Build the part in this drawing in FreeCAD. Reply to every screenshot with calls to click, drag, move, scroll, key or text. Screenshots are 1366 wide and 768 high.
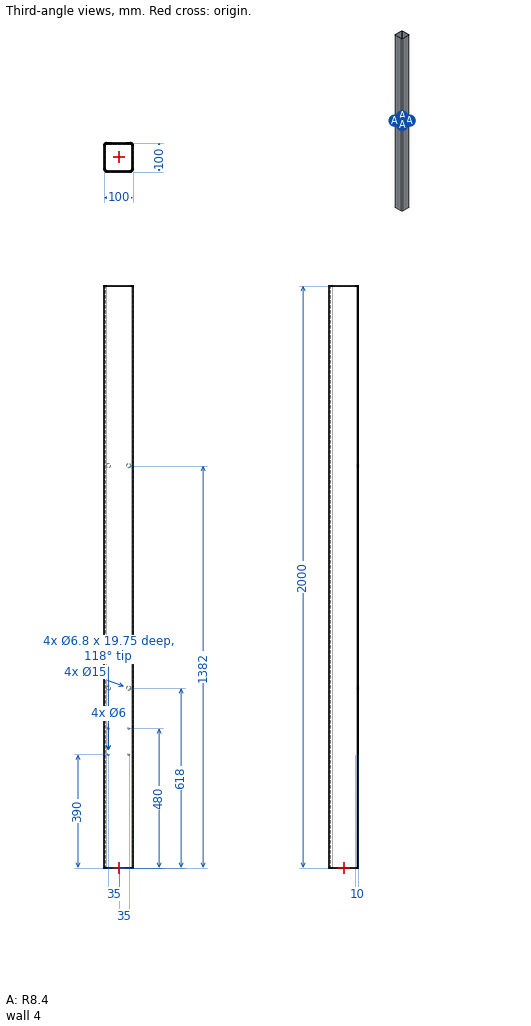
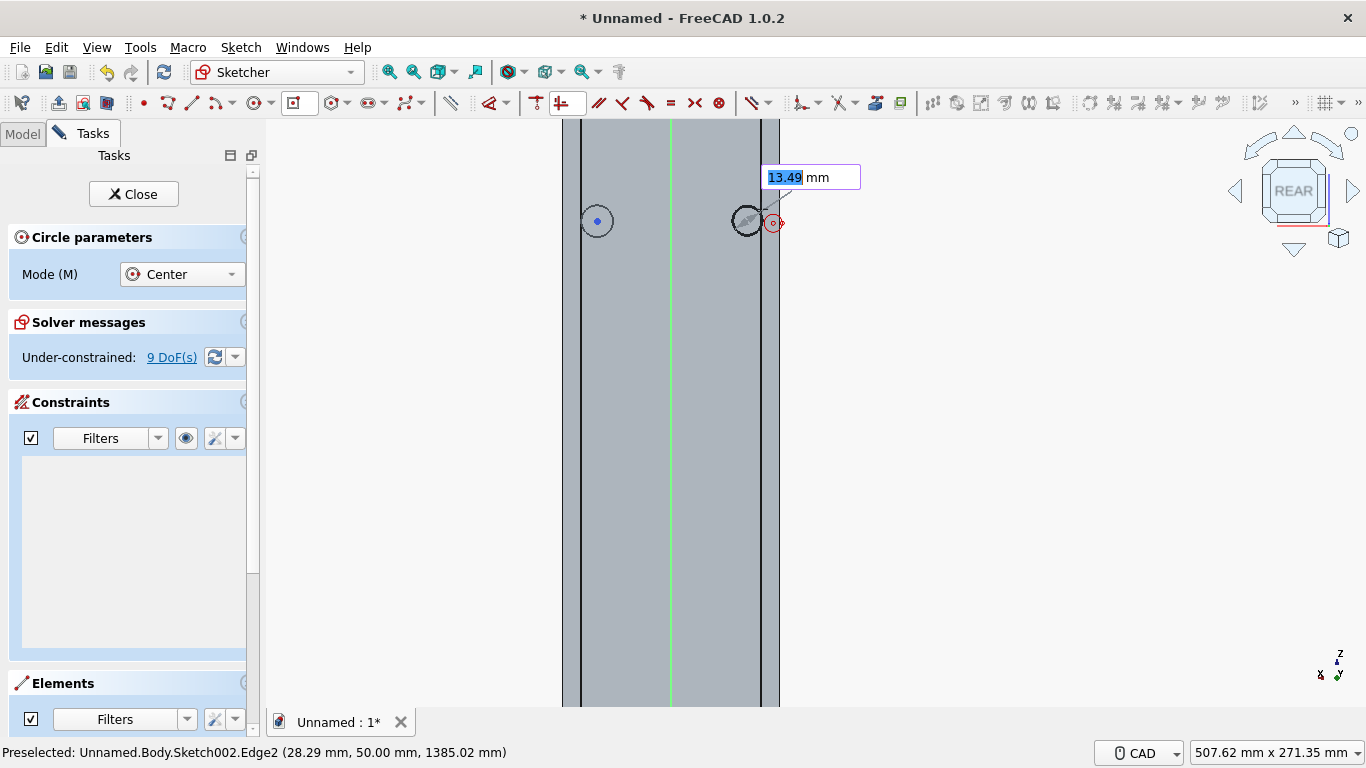
click(758, 207)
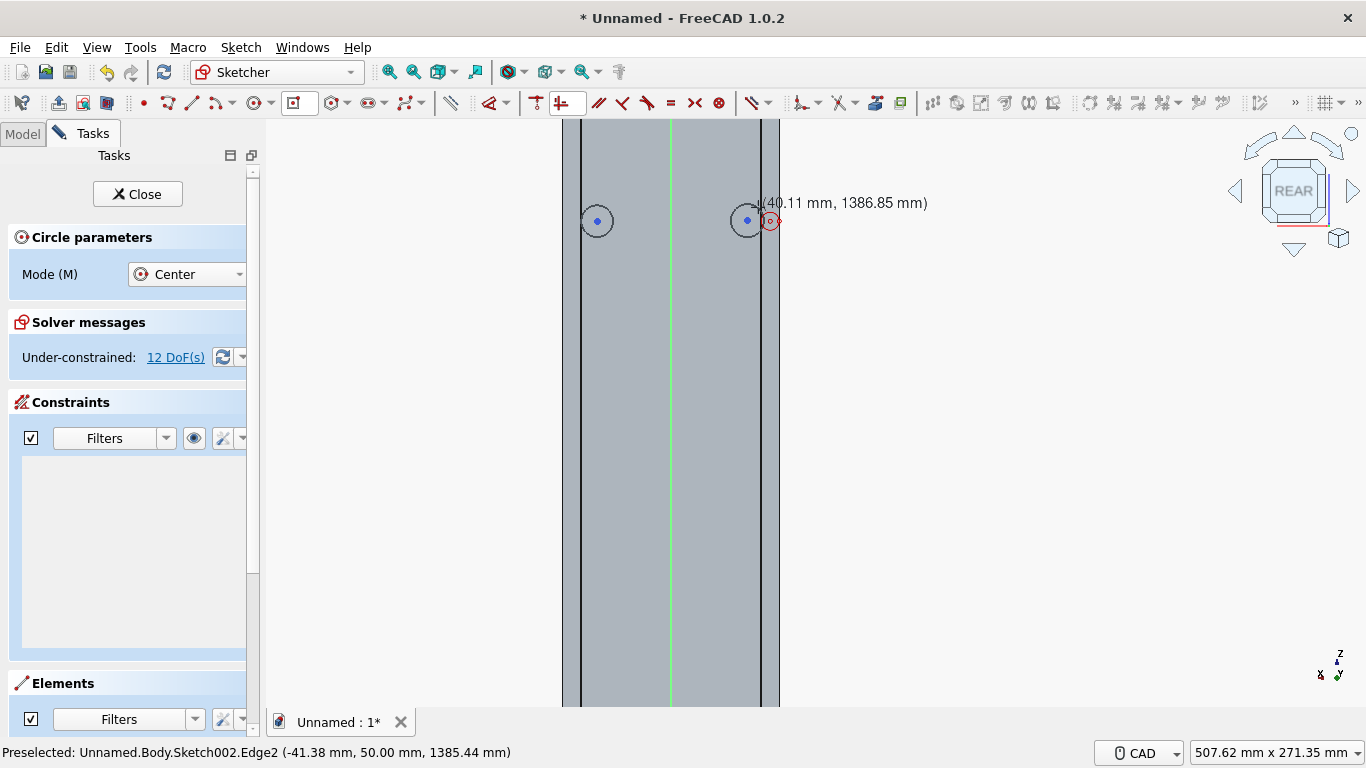
scroll(759, 210, down, 10)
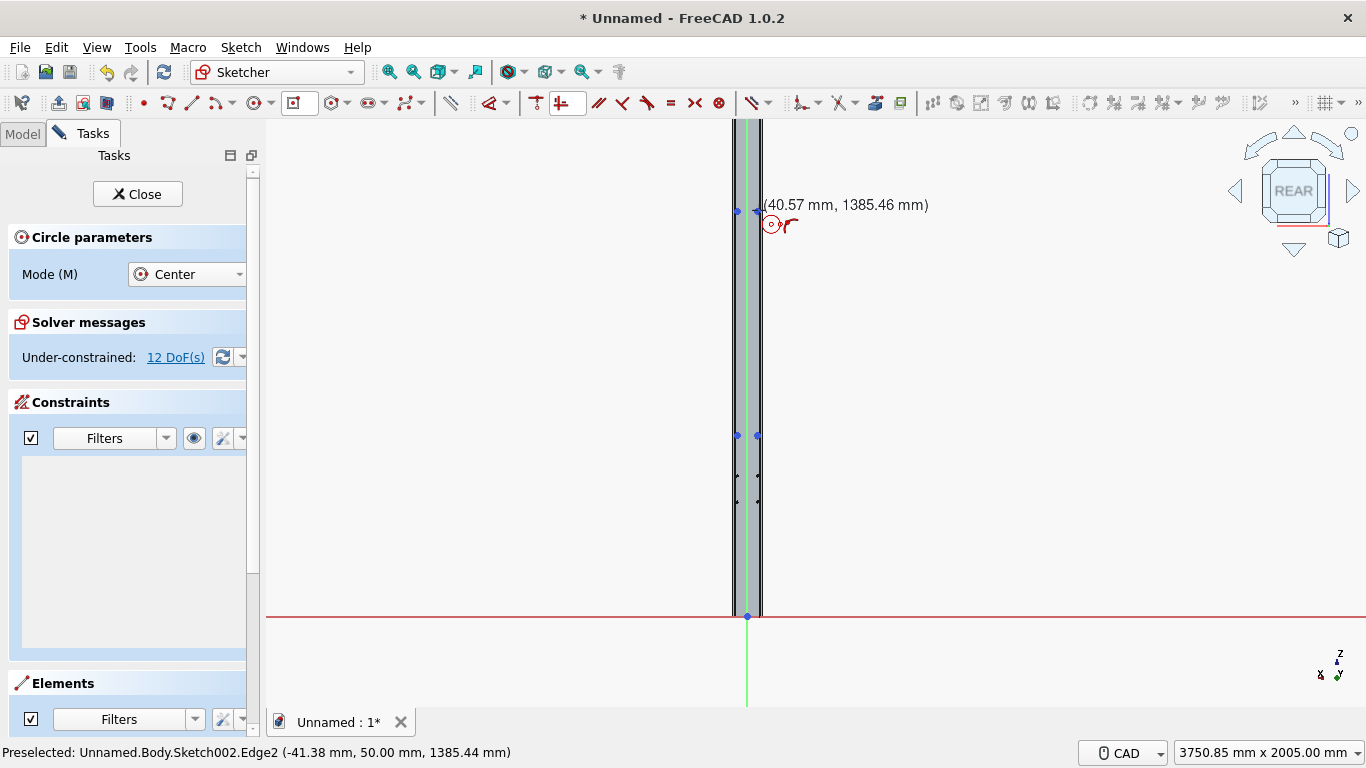
scroll(758, 502, up, 17)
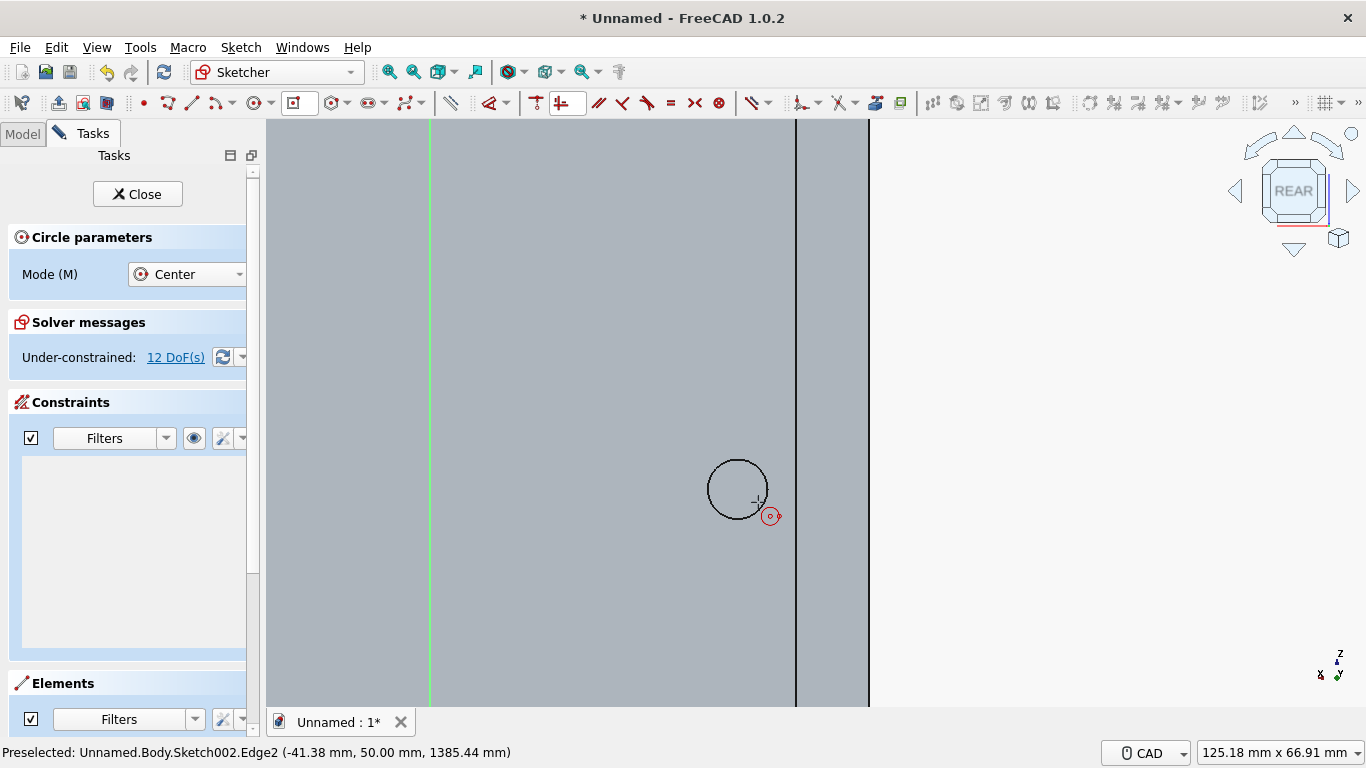
scroll(758, 503, down, 17)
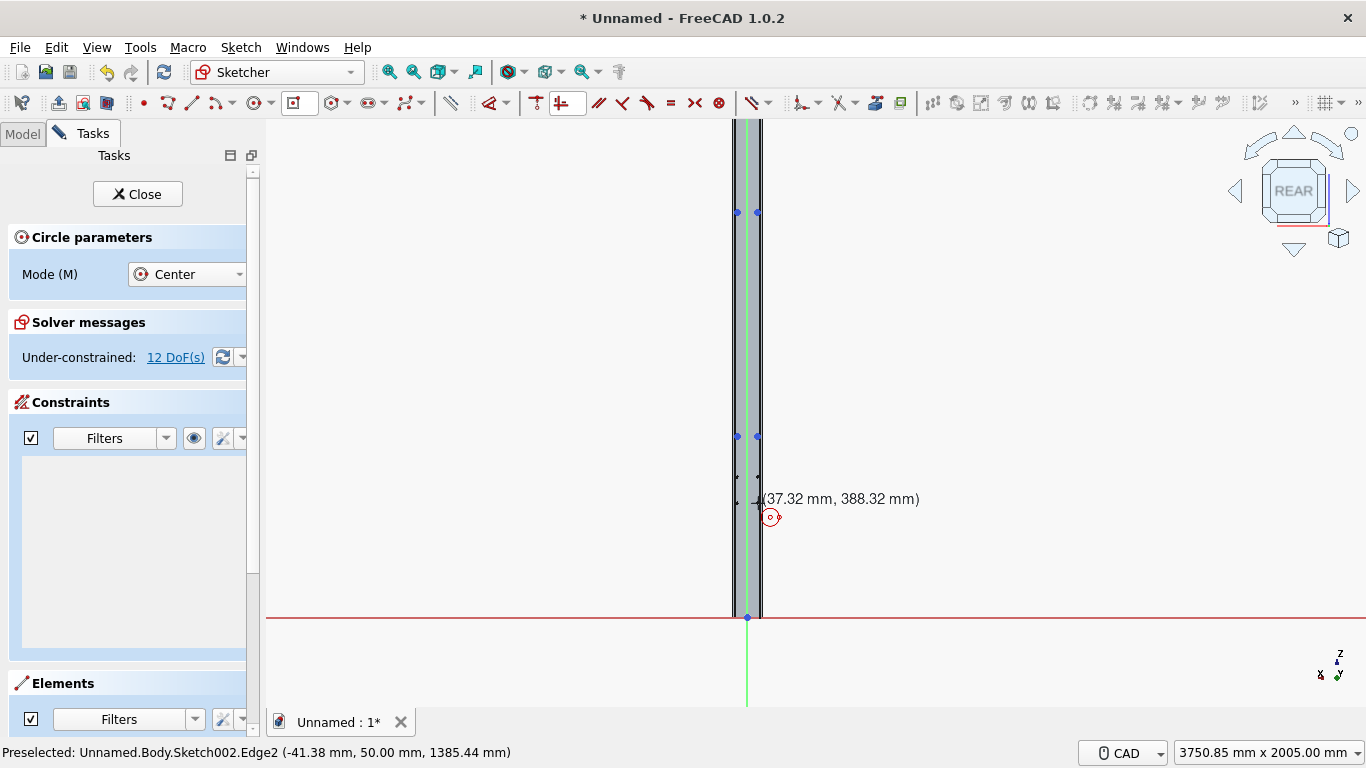
scroll(758, 503, up, 3)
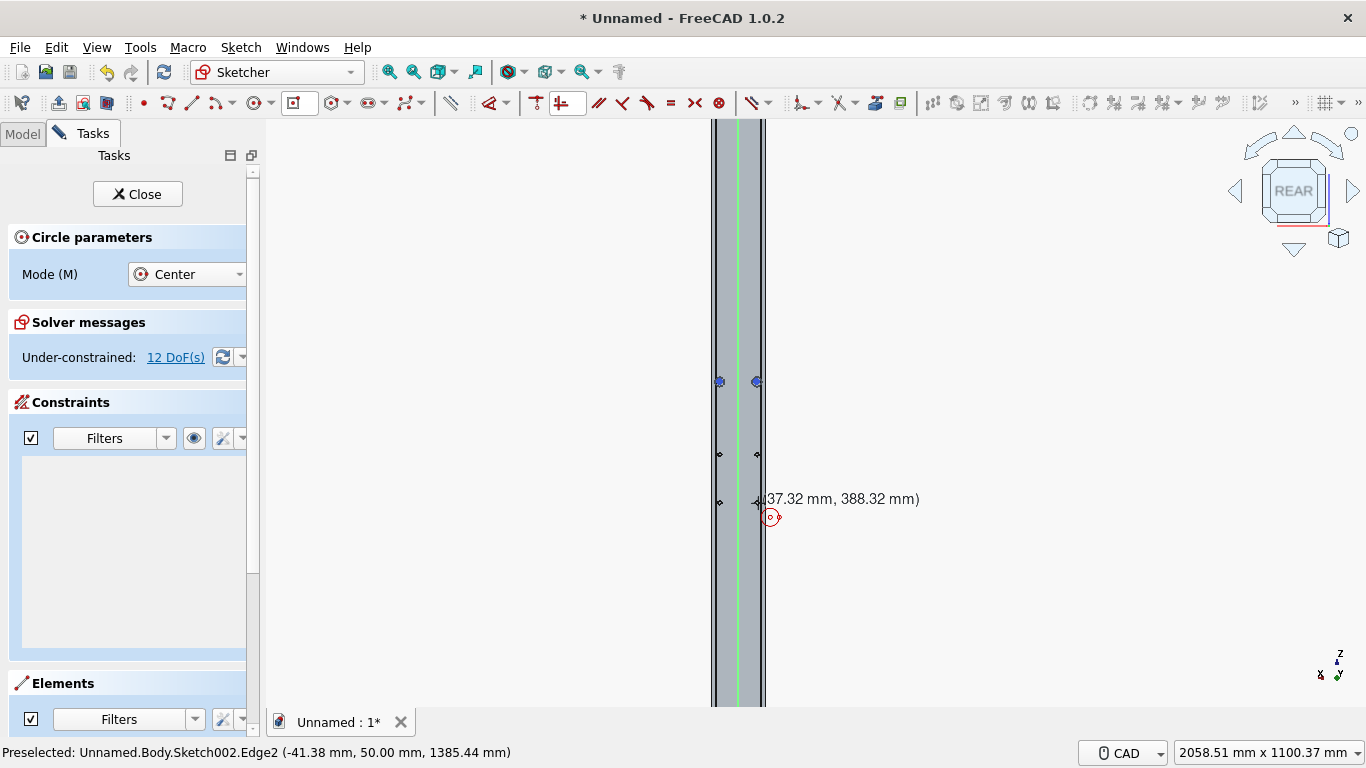
click(757, 503)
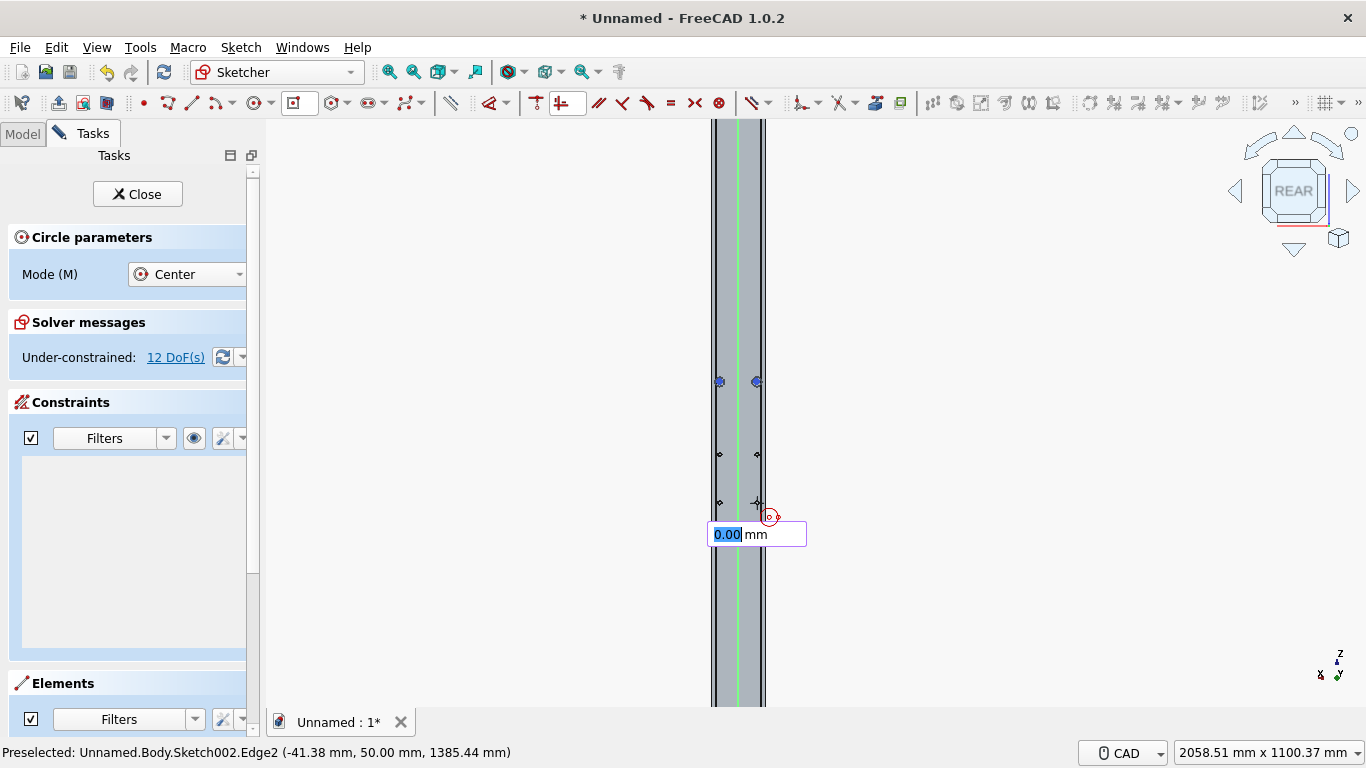
scroll(758, 502, up, 12)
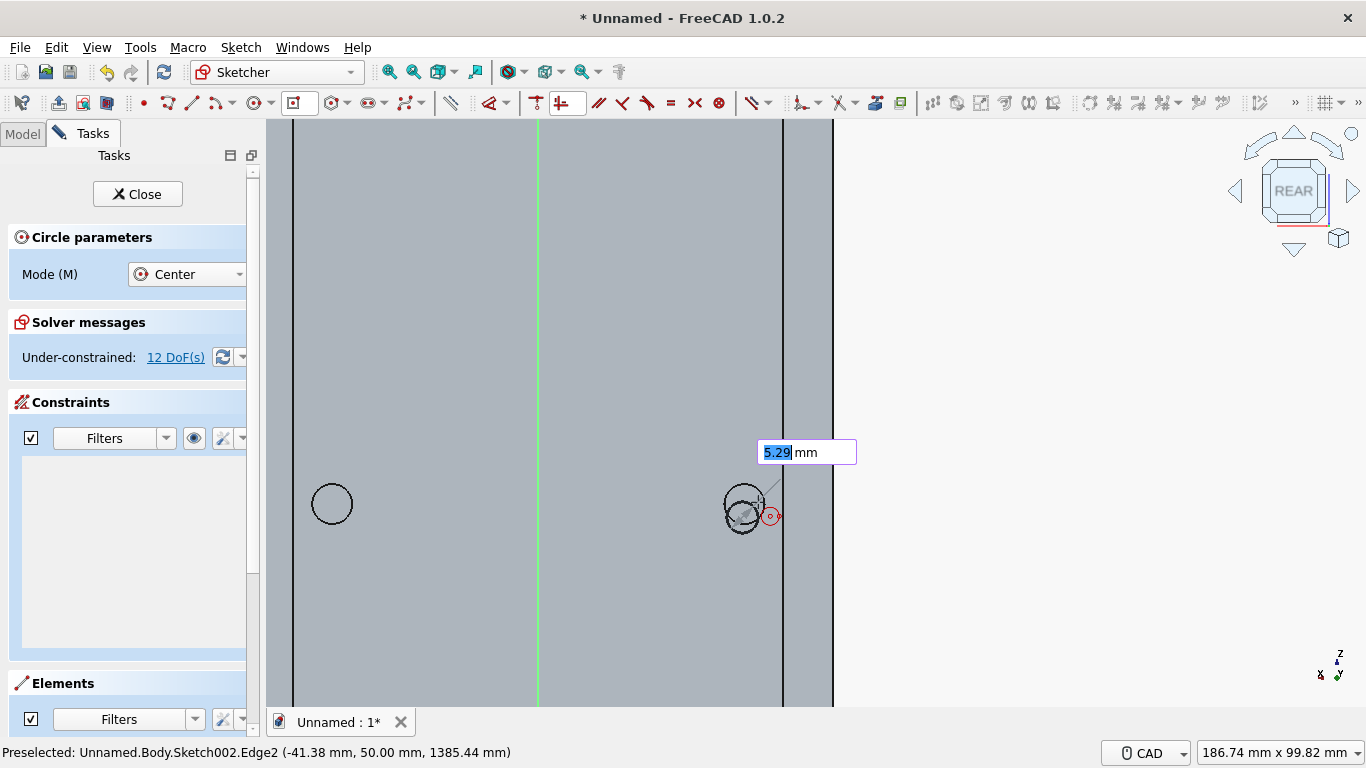
click(757, 492)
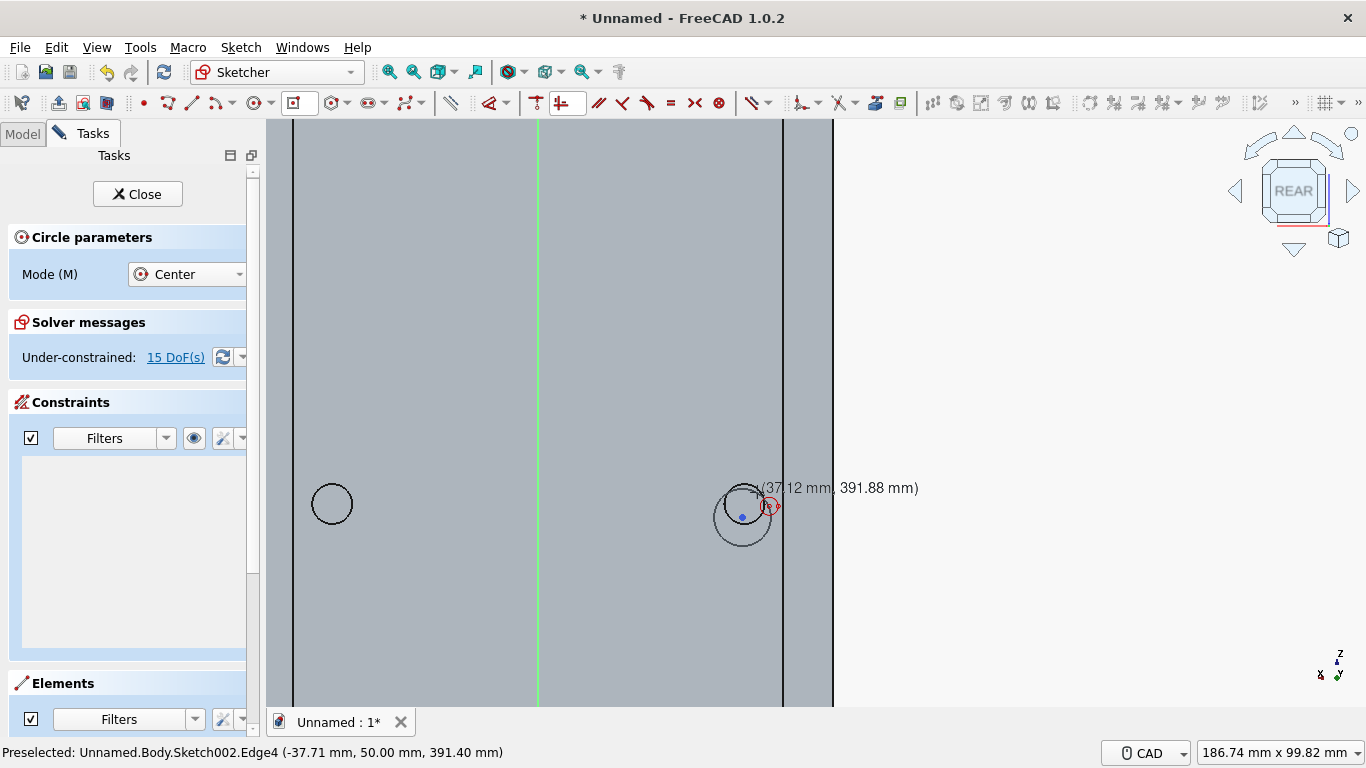
scroll(332, 504, up, 2)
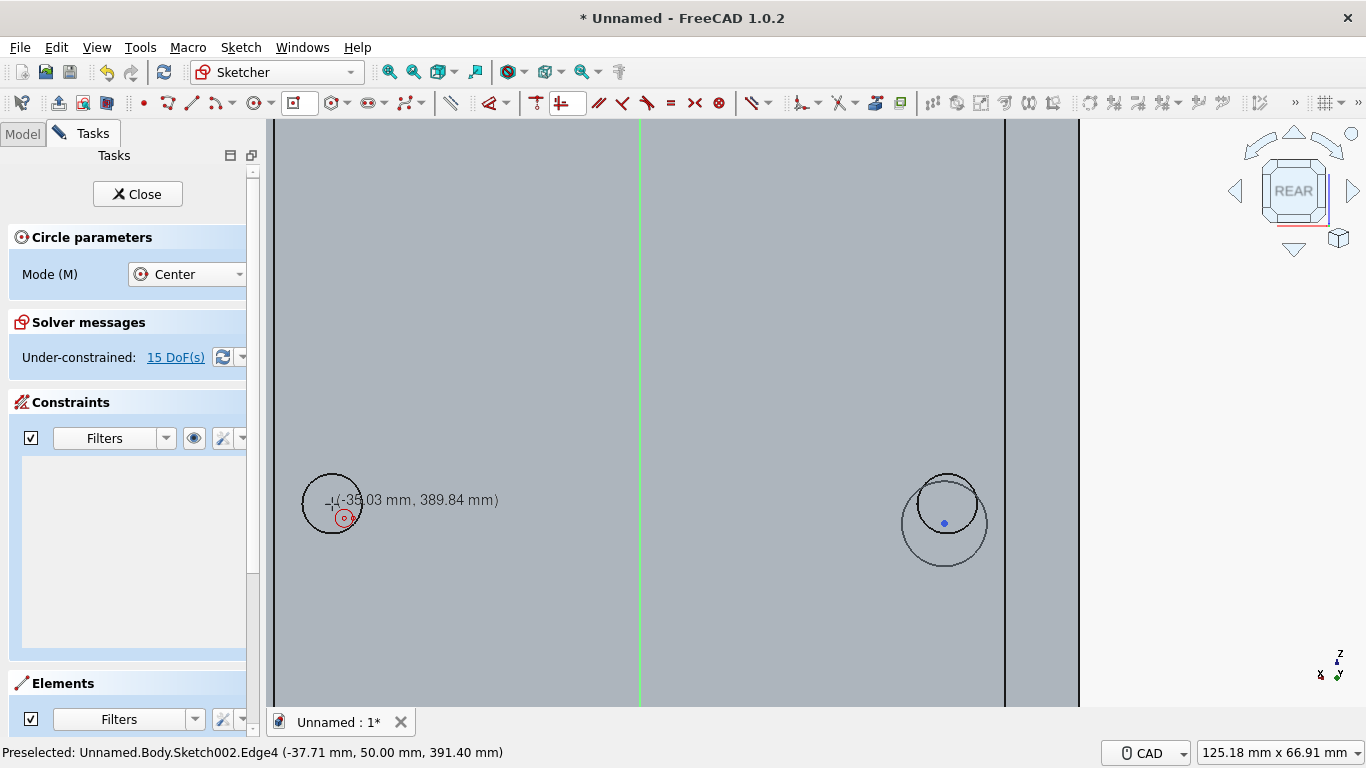
scroll(751, 502, down, 17)